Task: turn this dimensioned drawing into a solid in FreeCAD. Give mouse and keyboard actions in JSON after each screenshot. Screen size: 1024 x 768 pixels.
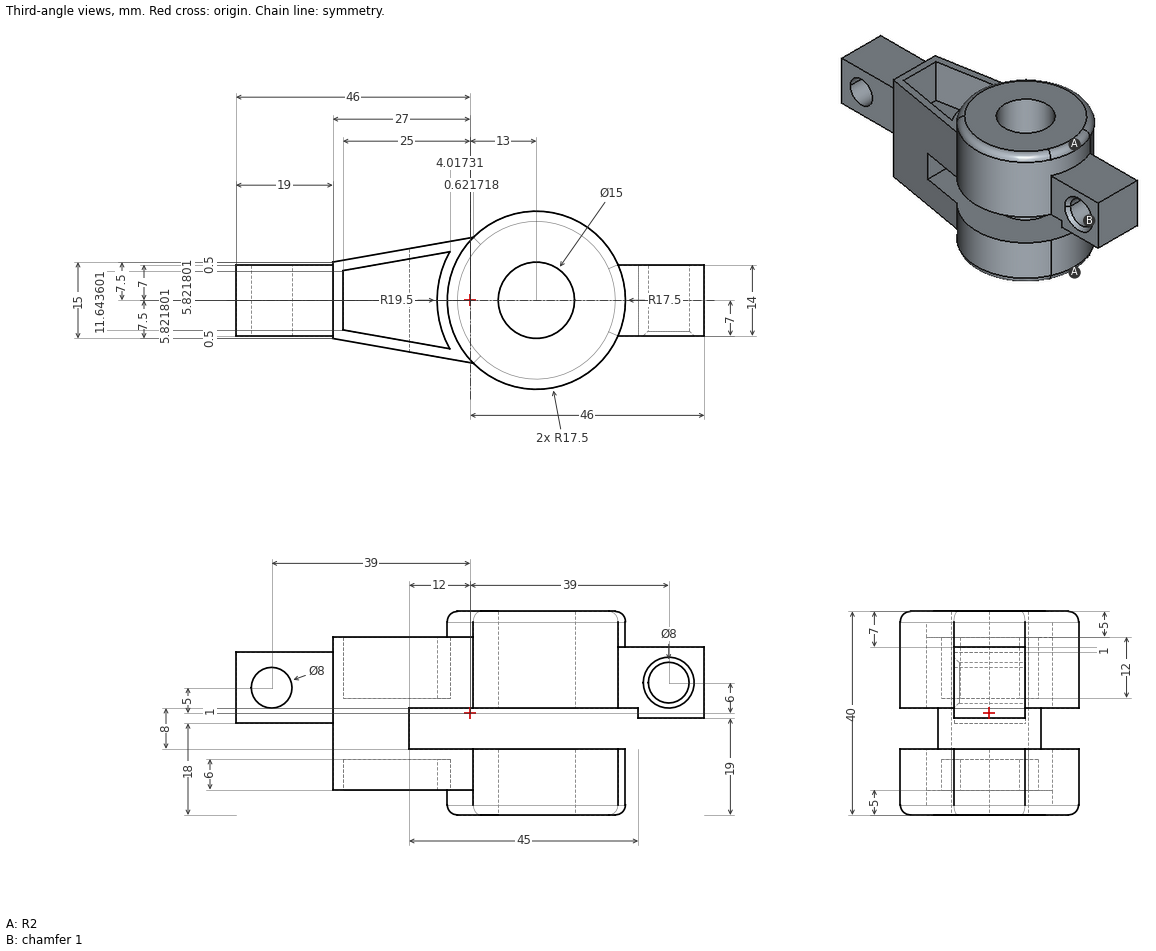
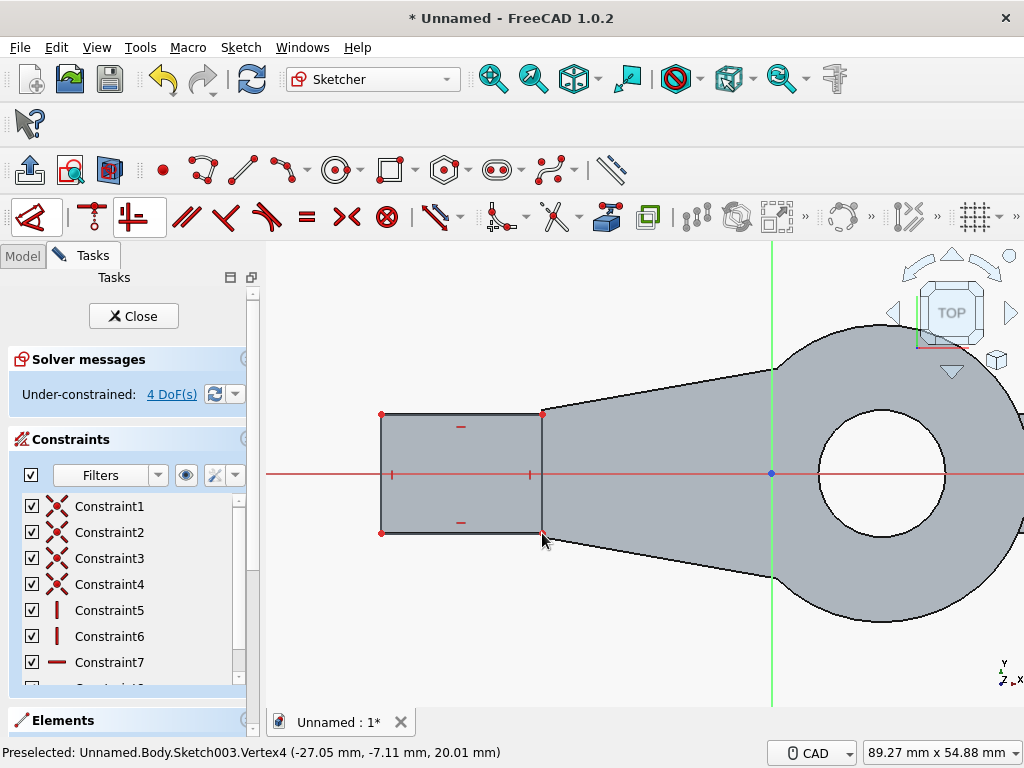
{"action": "left_click", "coordinate": [381, 451]}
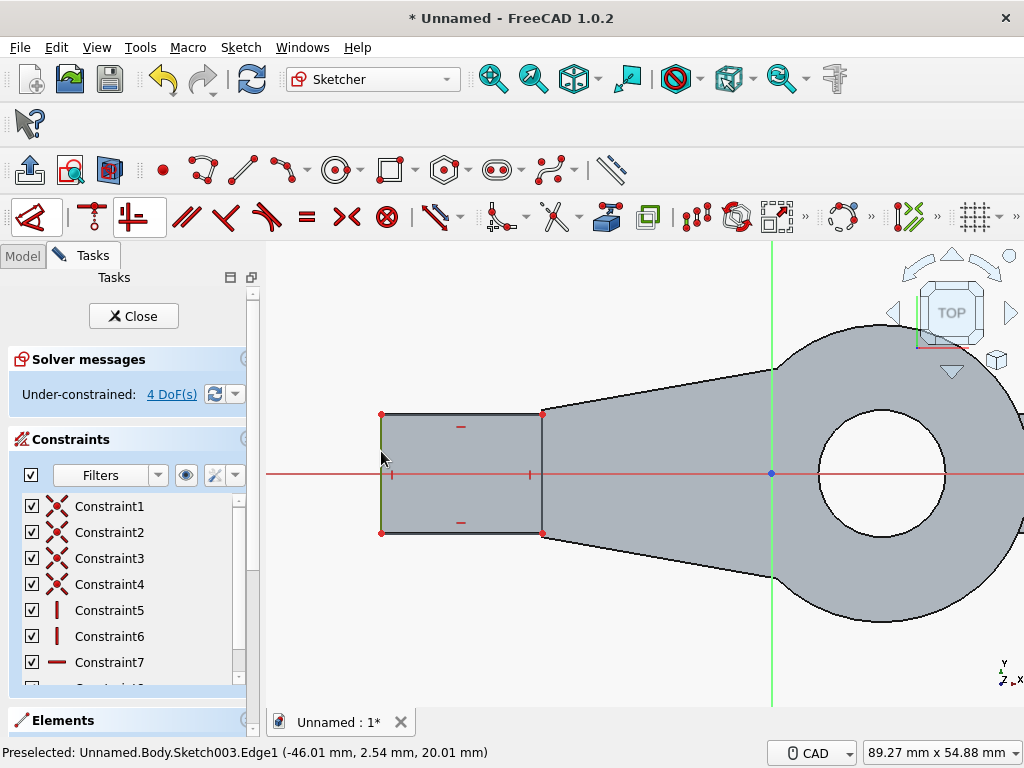
{"action": "left_click", "coordinate": [56, 218]}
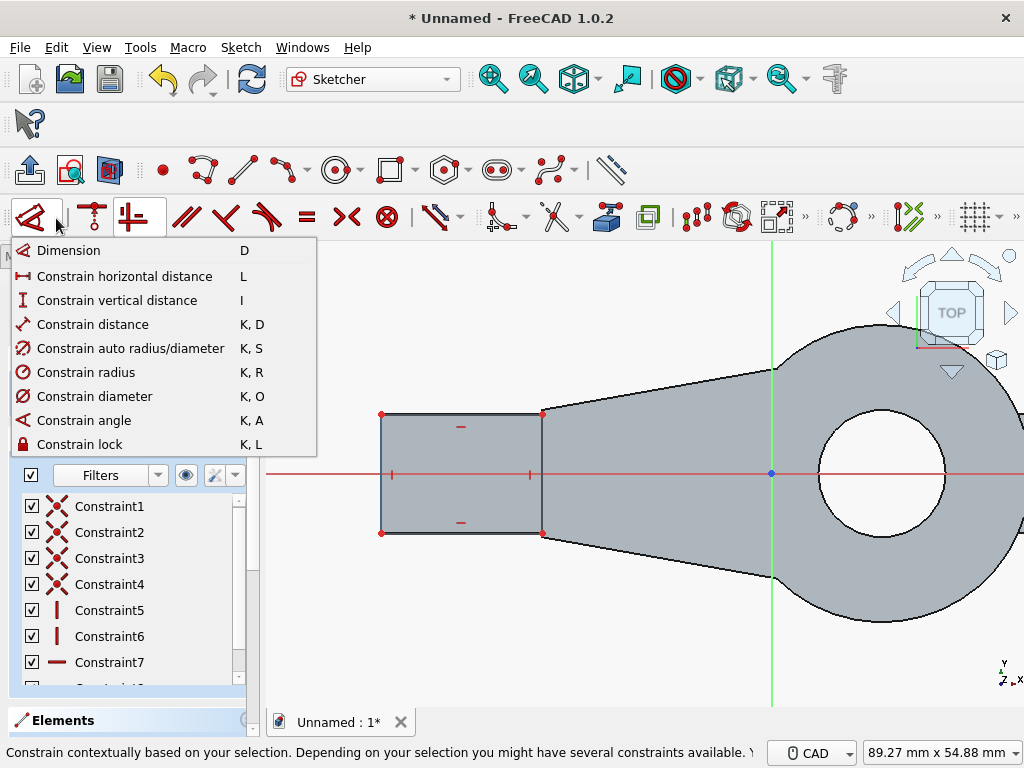
{"action": "left_click", "coordinate": [164, 300]}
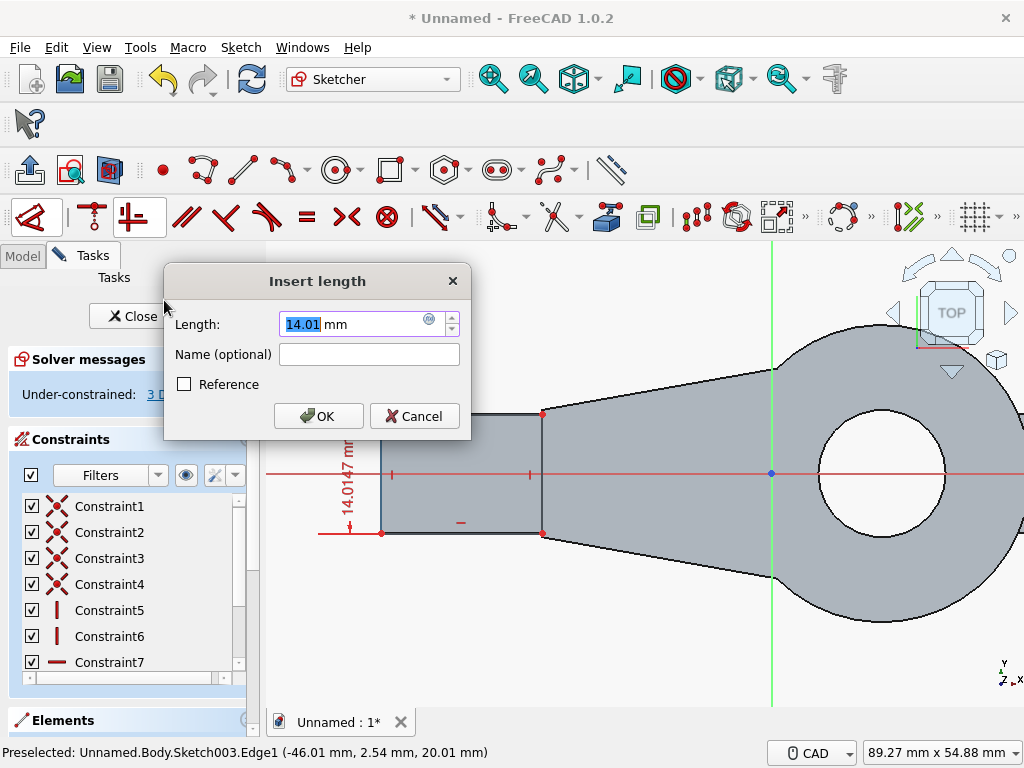
{"action": "type", "text": "14"}
{"action": "key", "text": "Return"}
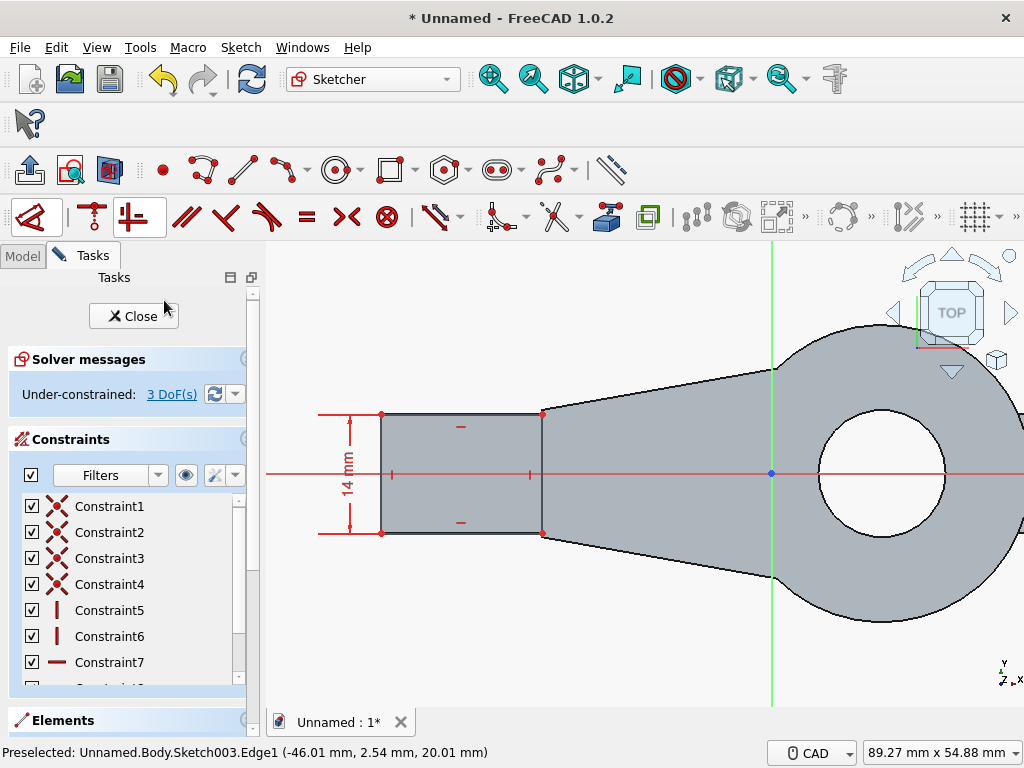
{"action": "left_click", "coordinate": [429, 534]}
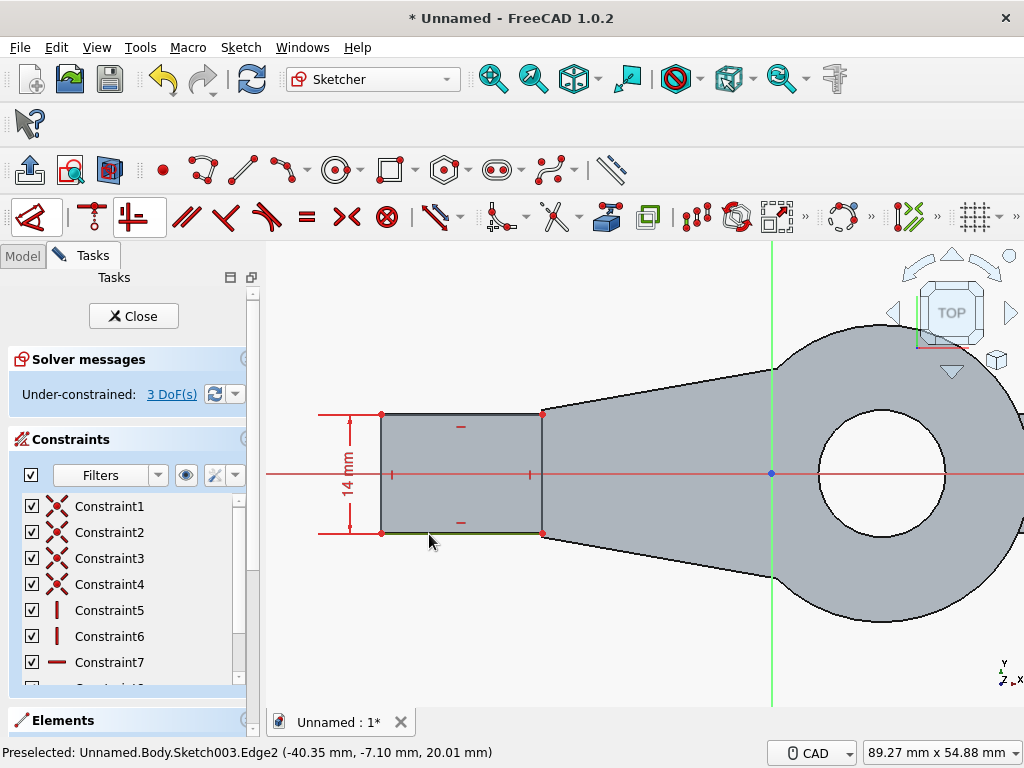
{"action": "left_click", "coordinate": [56, 218]}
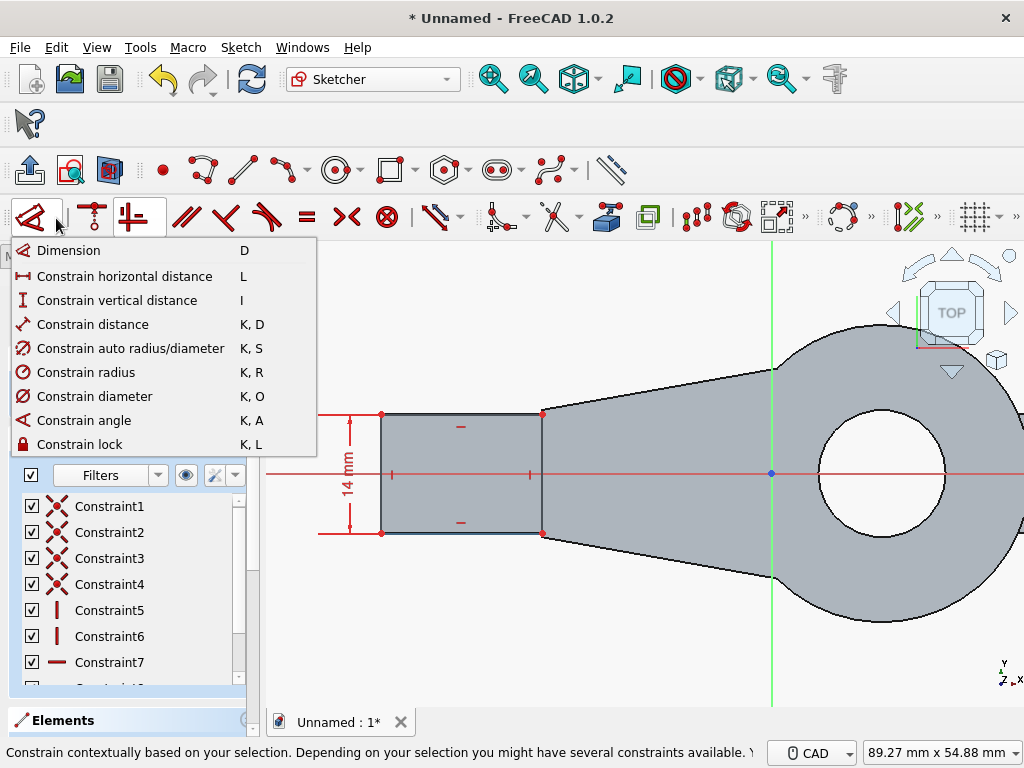
{"action": "left_click", "coordinate": [164, 276]}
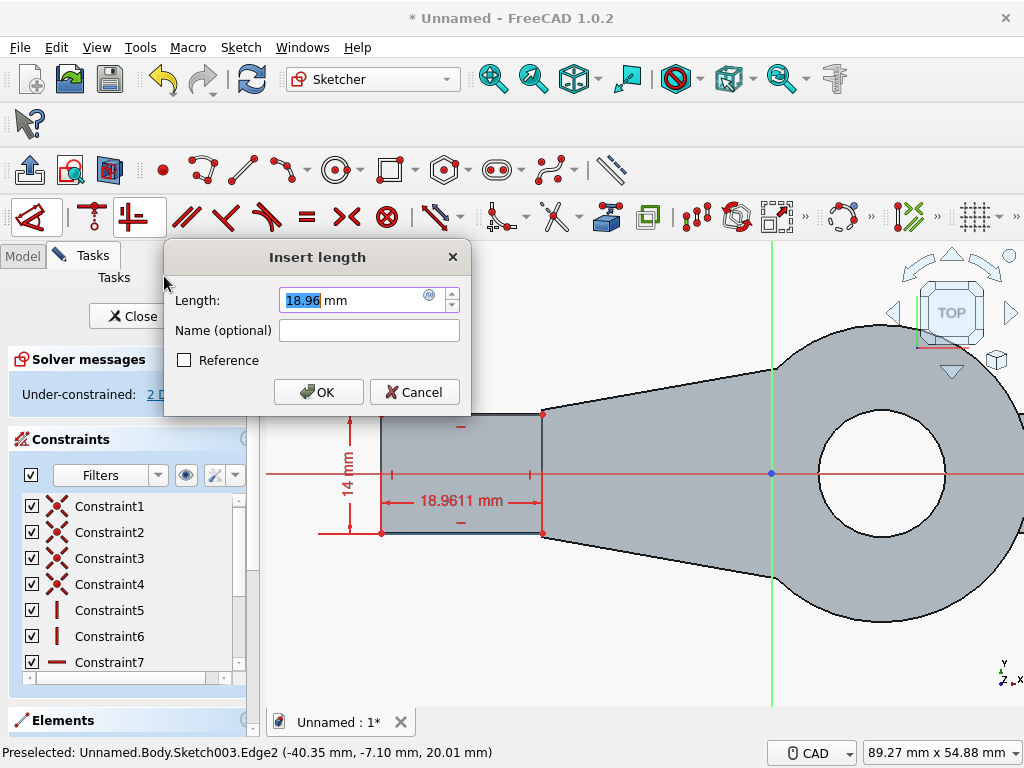
{"action": "type", "text": "19"}
{"action": "key", "text": "Return"}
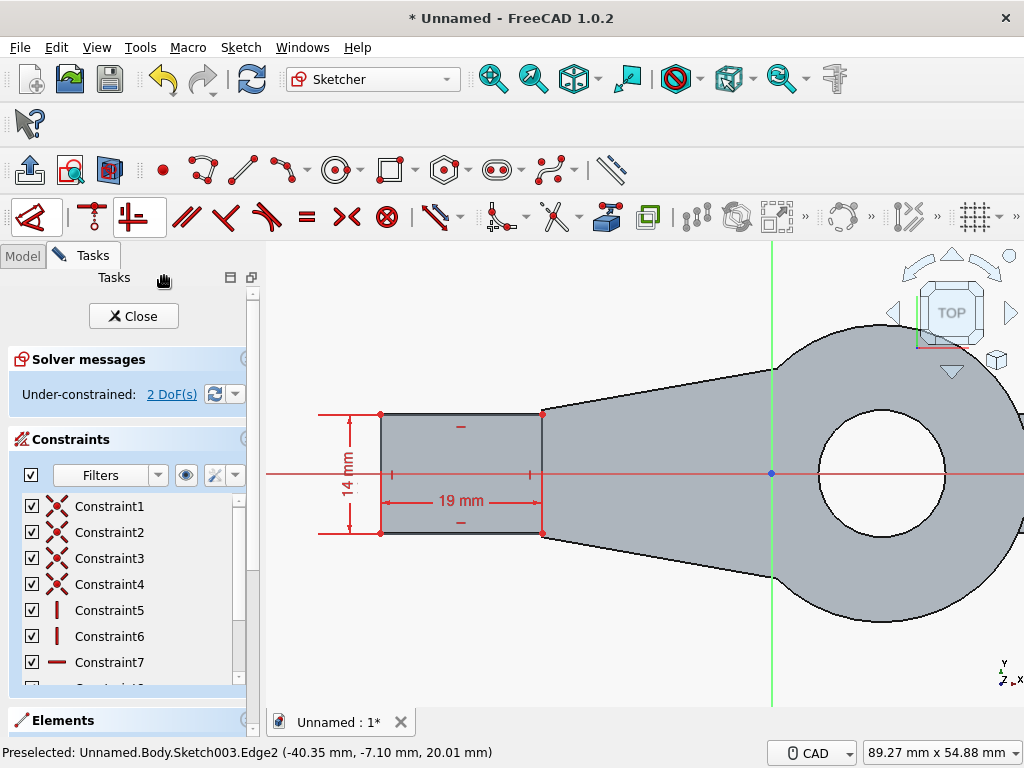
{"action": "left_click", "coordinate": [381, 415]}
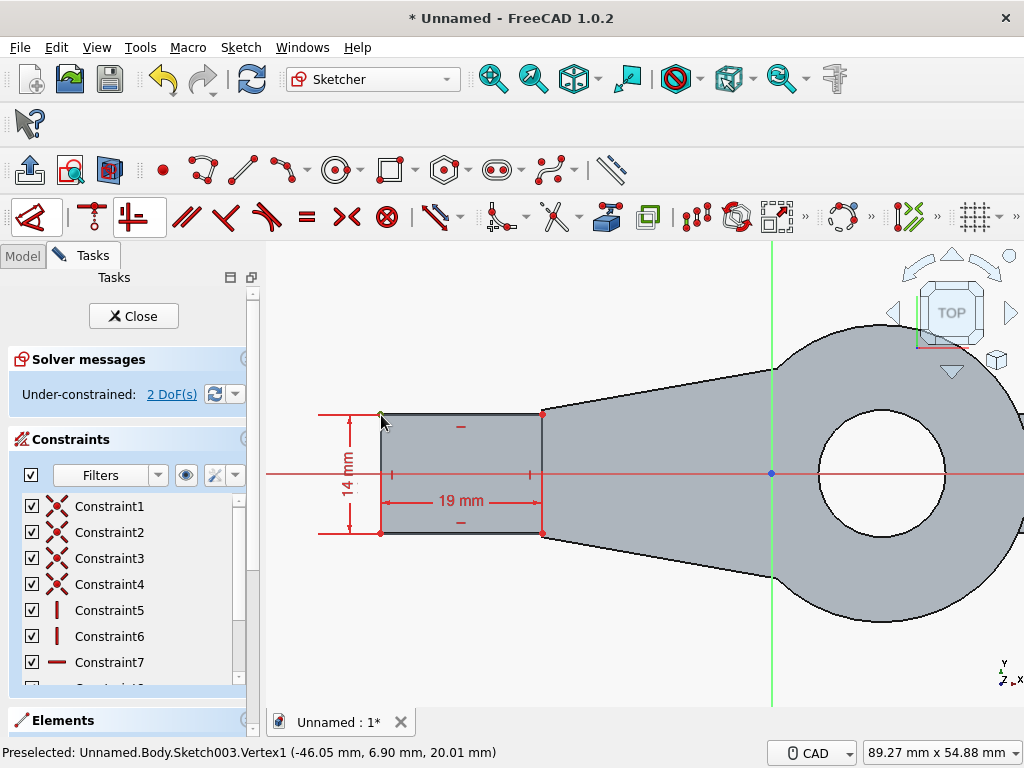
{"action": "key", "text": "i"}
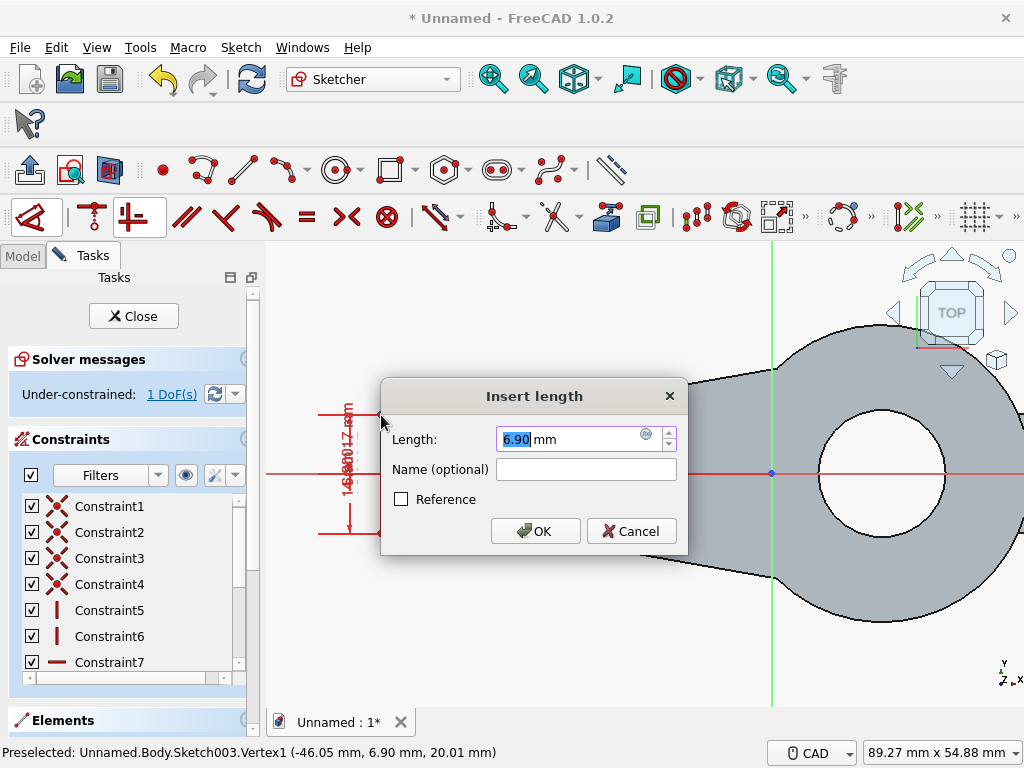
{"action": "type", "text": "7"}
{"action": "key", "text": "Return"}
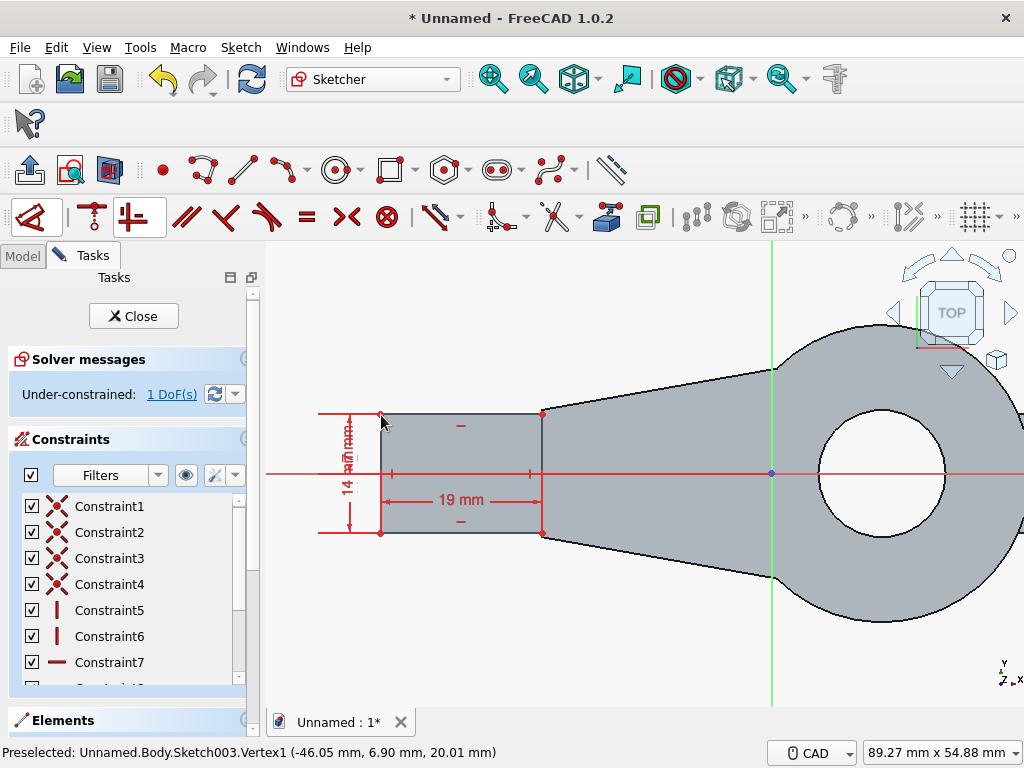
{"action": "left_click", "coordinate": [381, 414]}